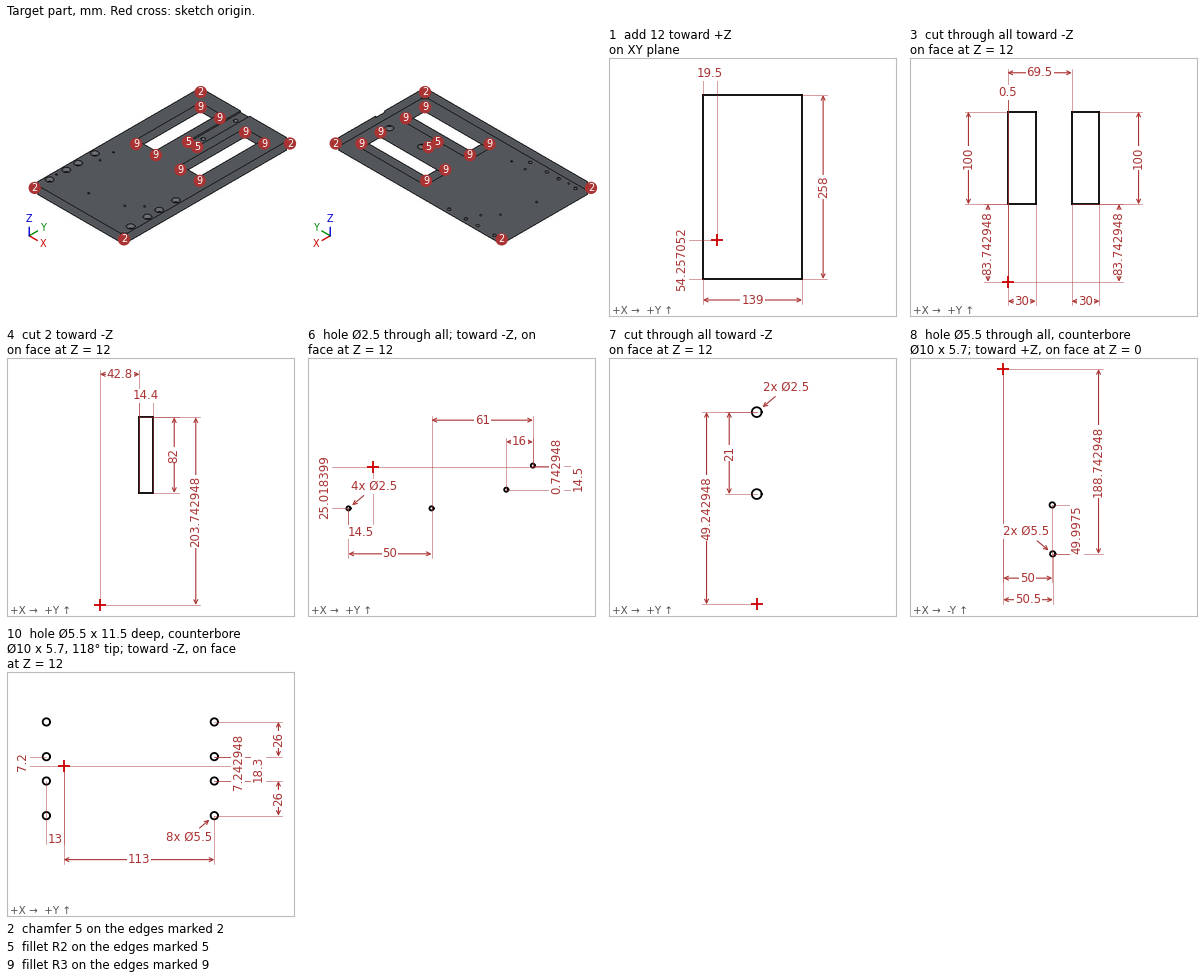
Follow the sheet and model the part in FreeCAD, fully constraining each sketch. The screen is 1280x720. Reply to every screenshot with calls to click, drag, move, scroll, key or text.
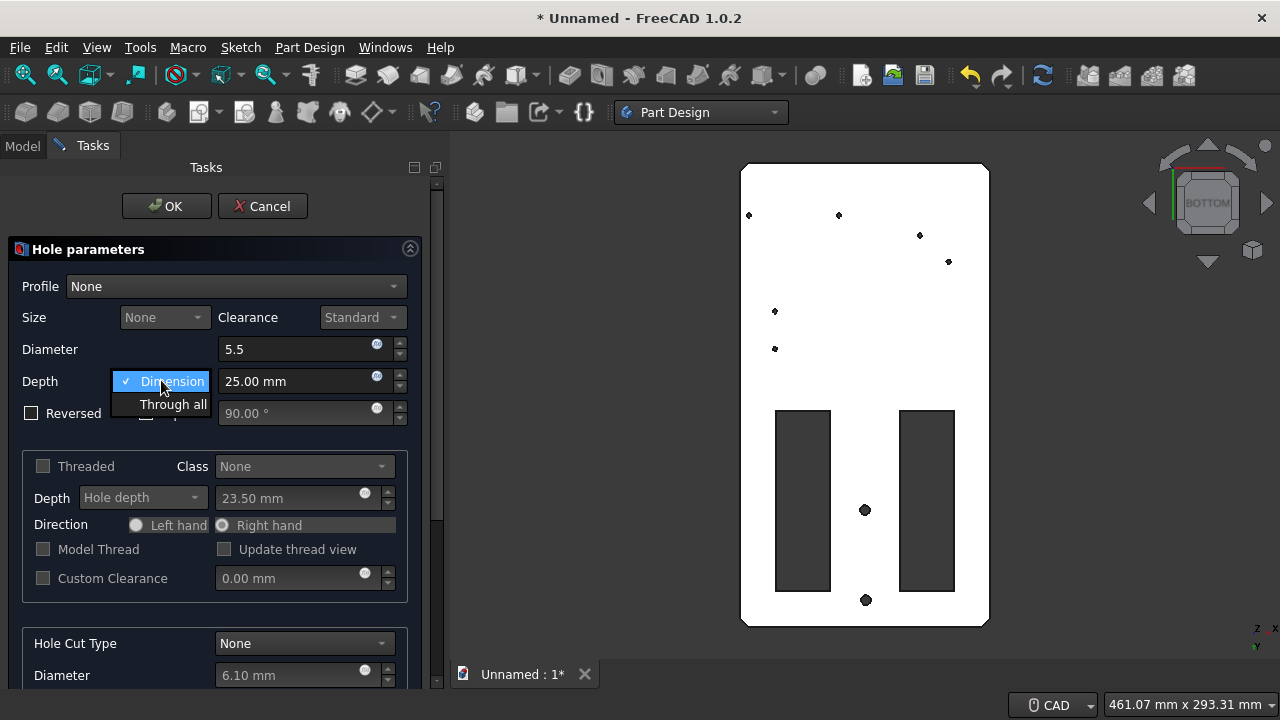
click(160, 404)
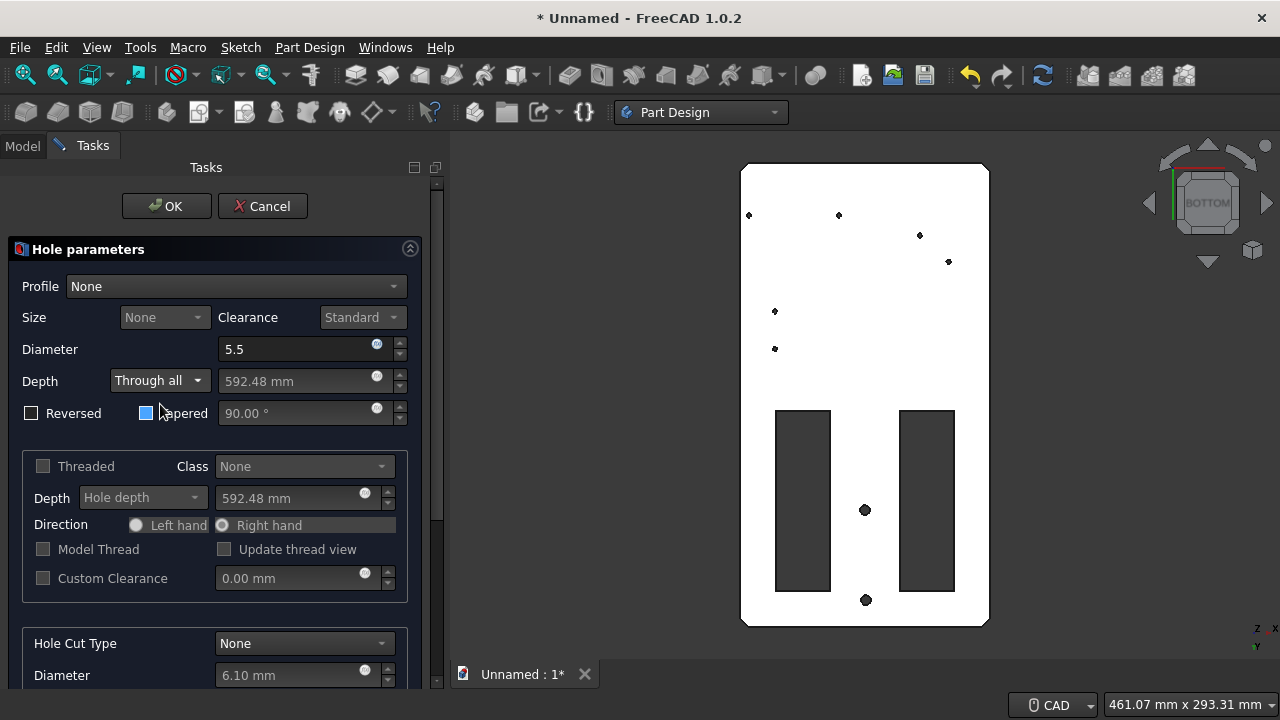
click(306, 644)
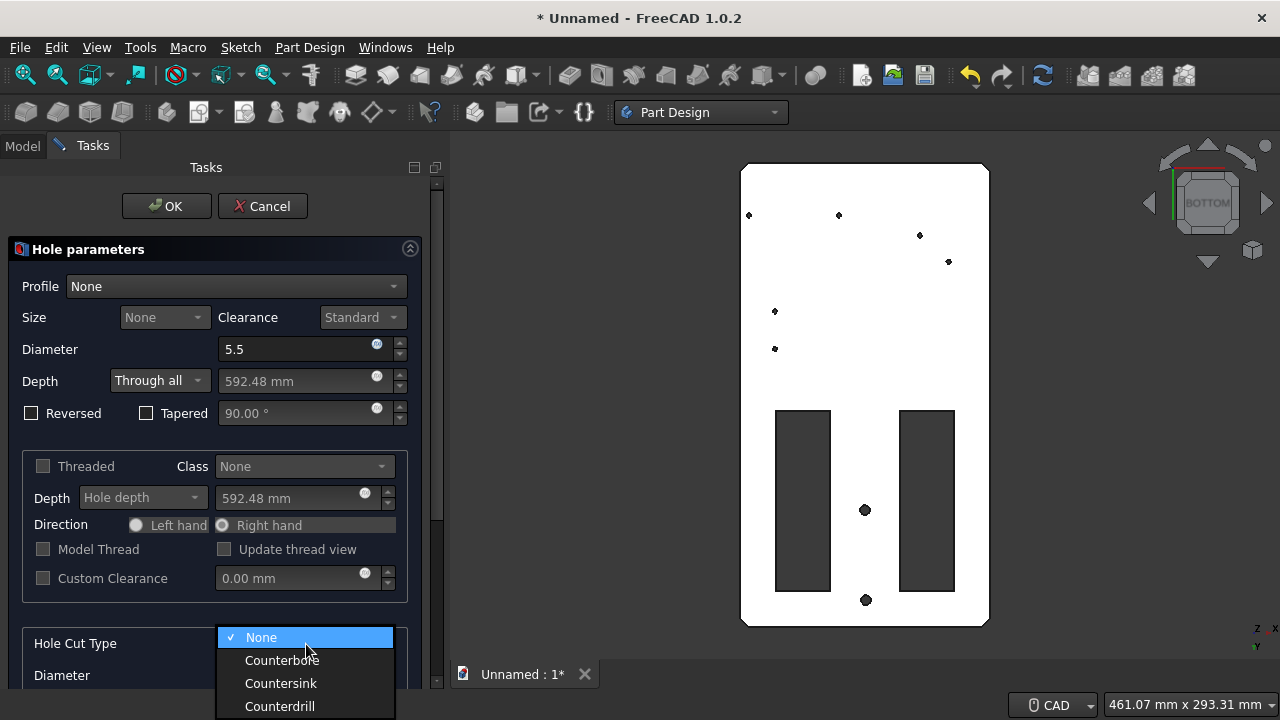
click(304, 660)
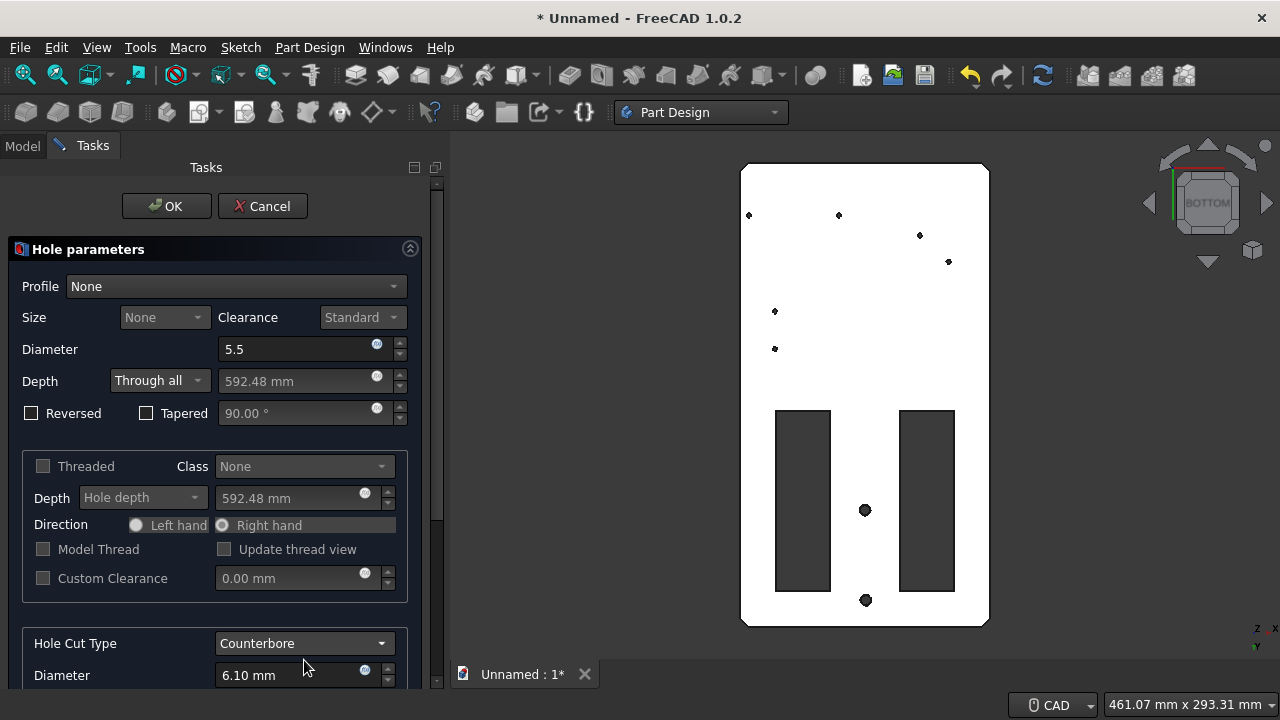
triple_click(298, 675)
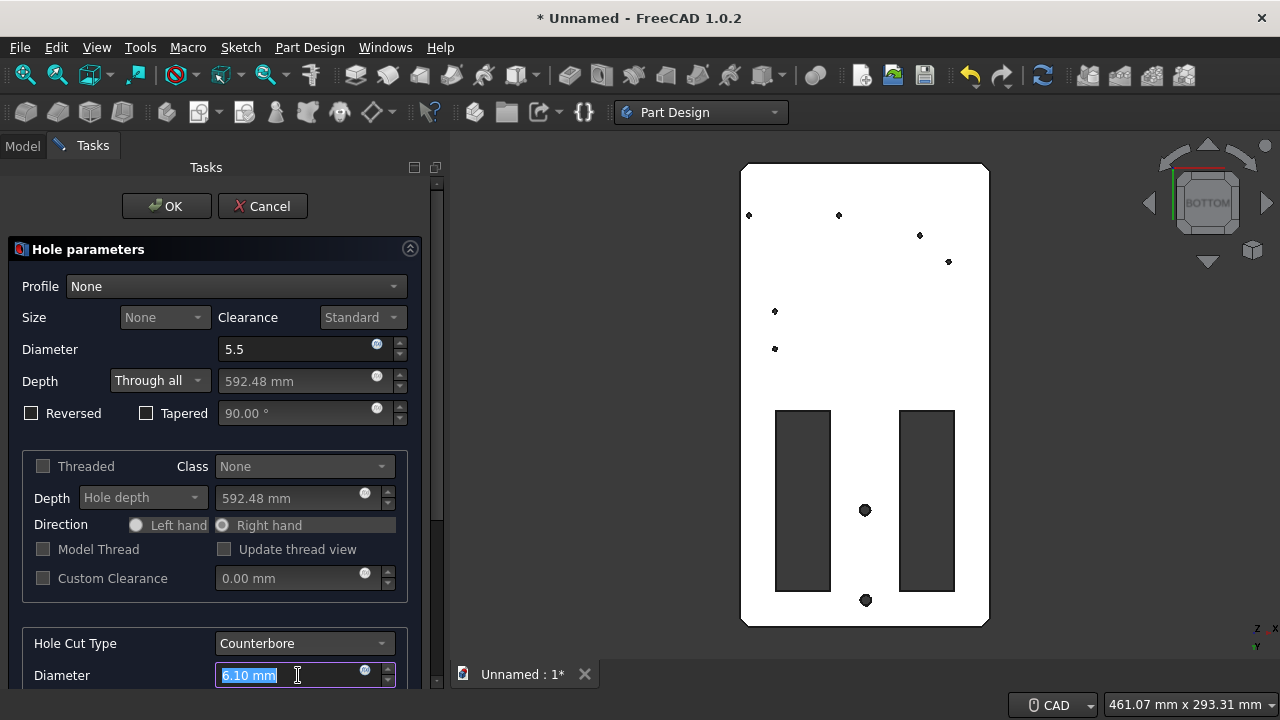
text(10)
key(Tab)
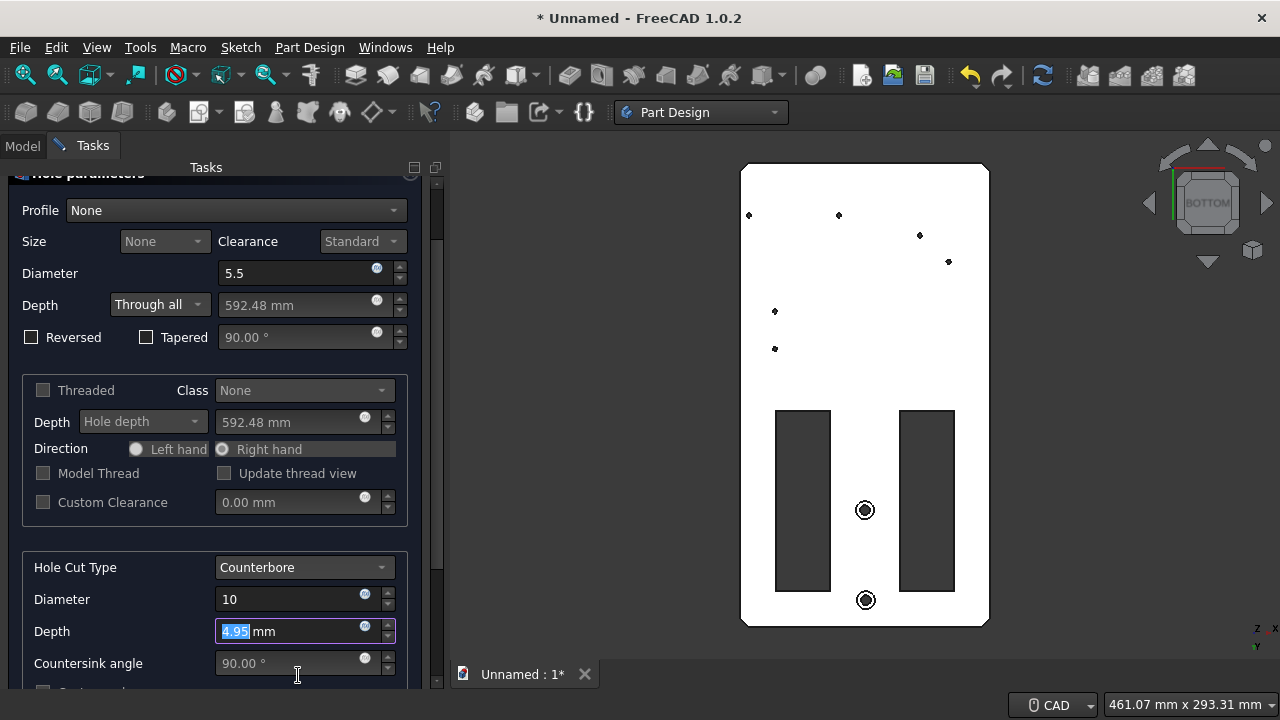
text(5.7)
key(Tab)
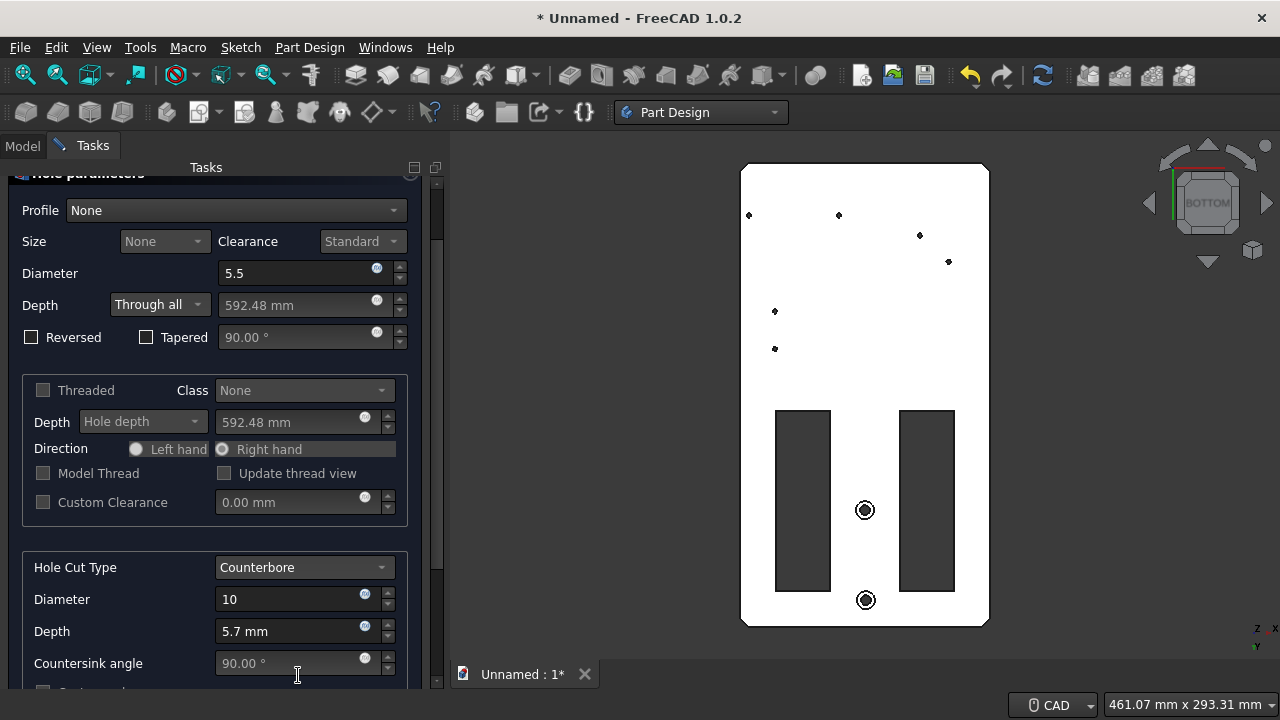
scroll(437, 432, up, 3)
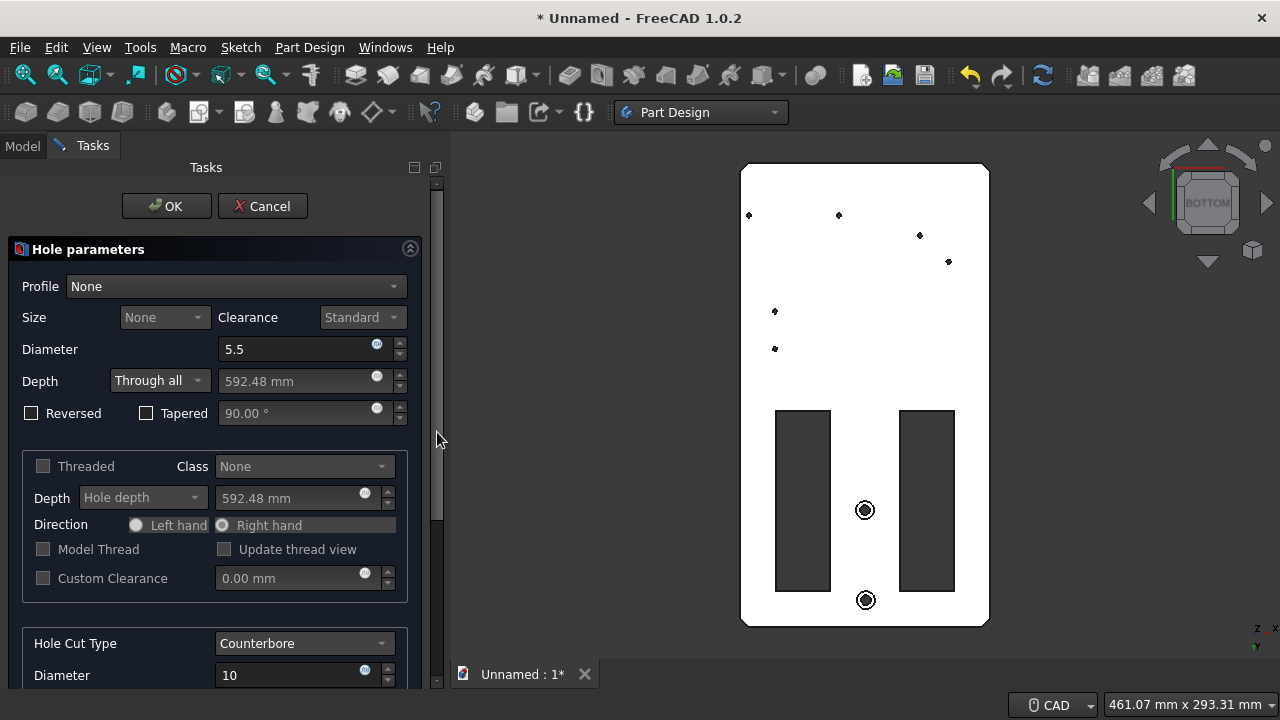
click(167, 206)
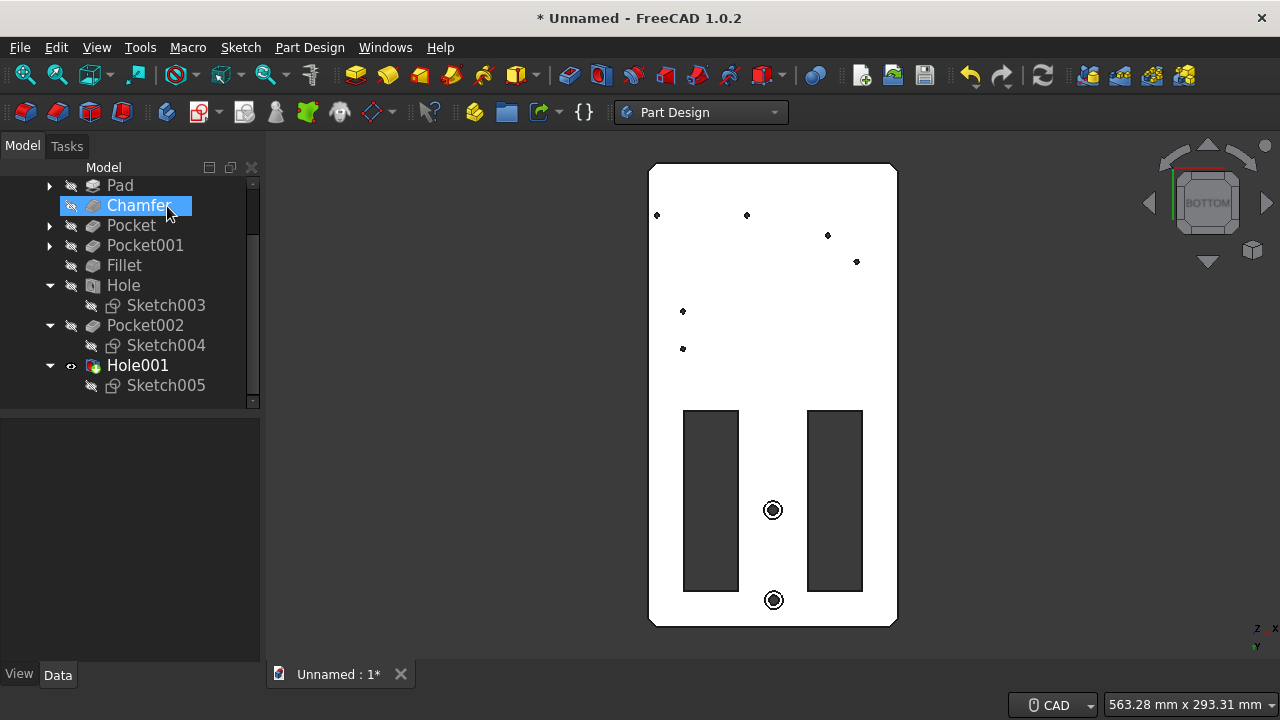
scroll(862, 590, up, 4)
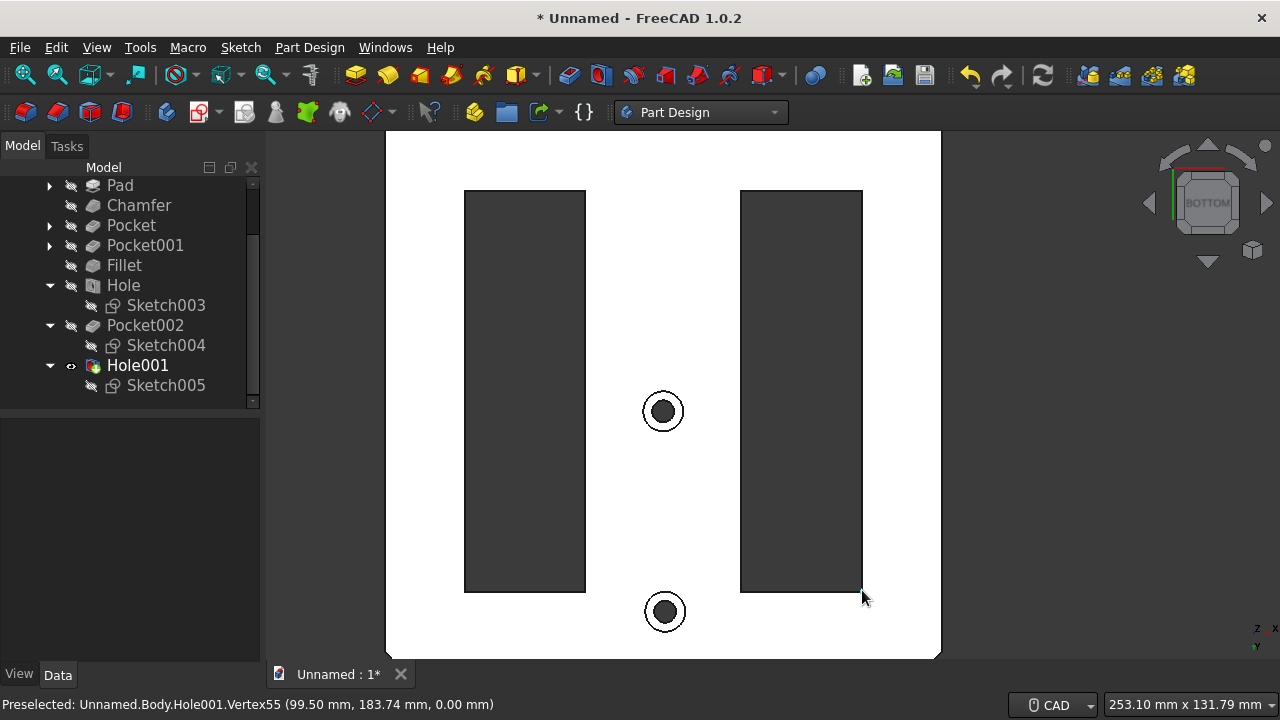
key(v)
key(f)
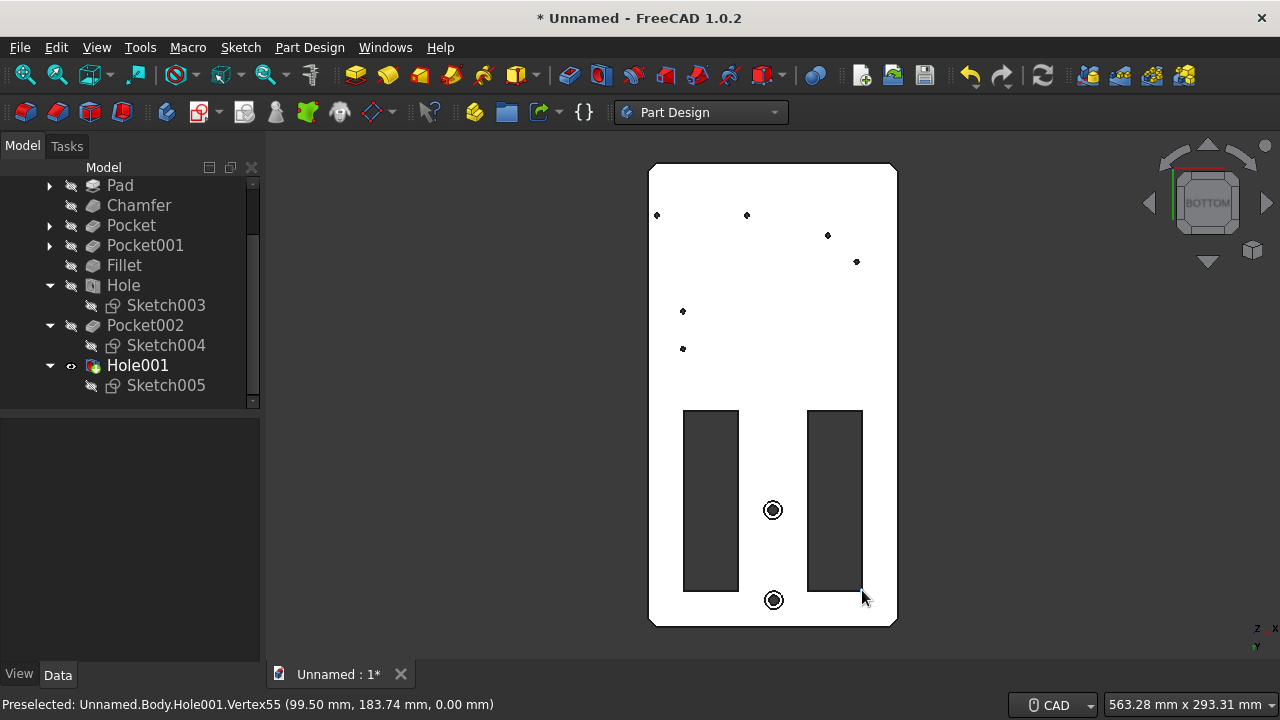
key(0)